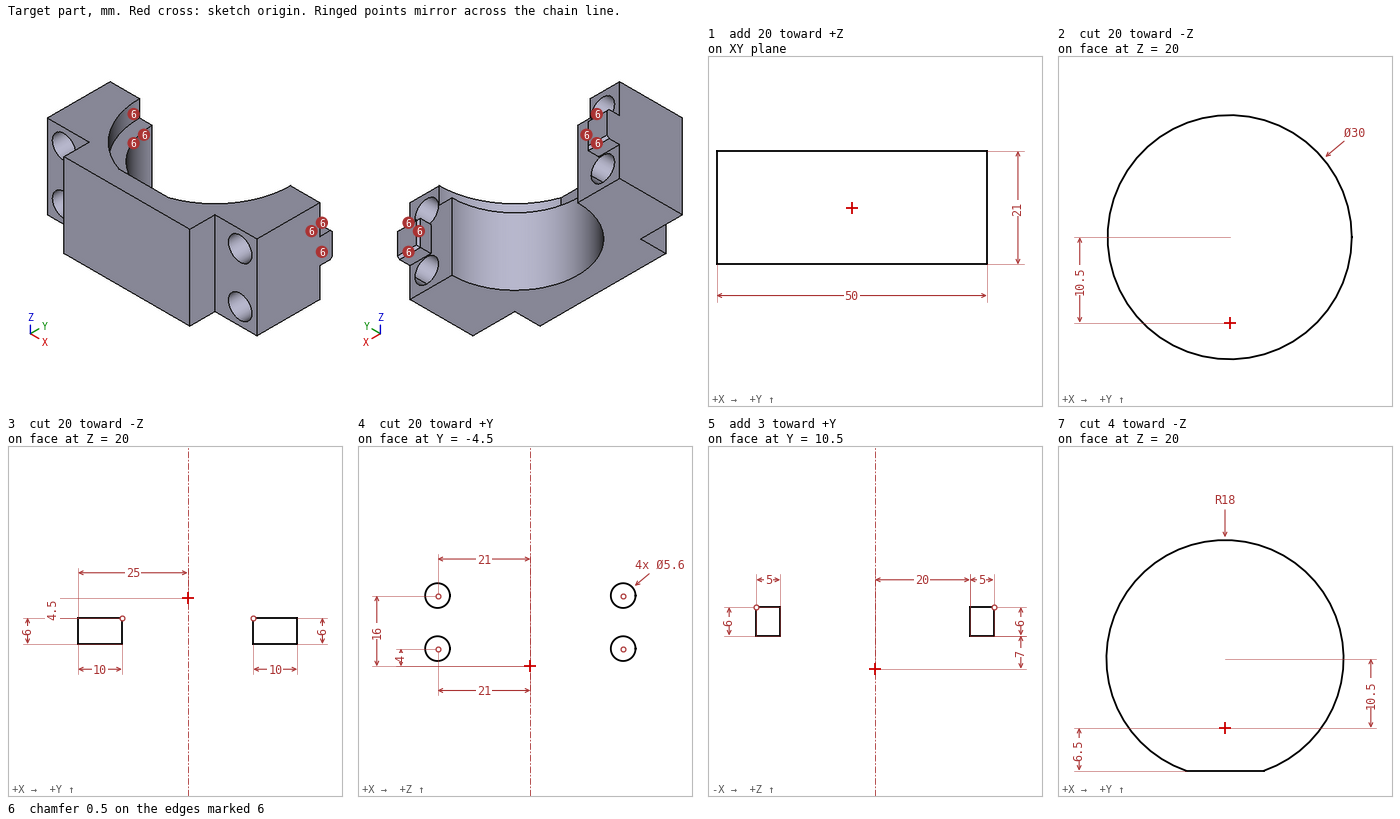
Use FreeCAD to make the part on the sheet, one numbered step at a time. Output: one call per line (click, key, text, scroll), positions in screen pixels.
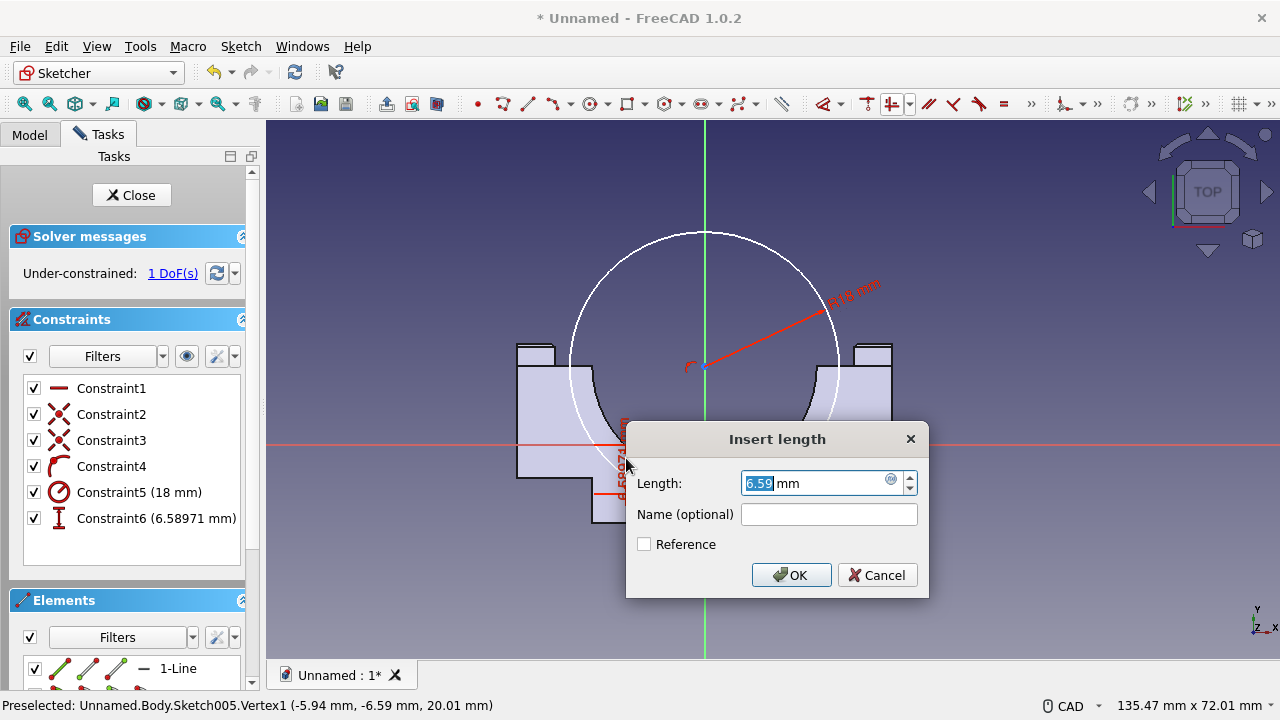
text(6.5)
key(Return)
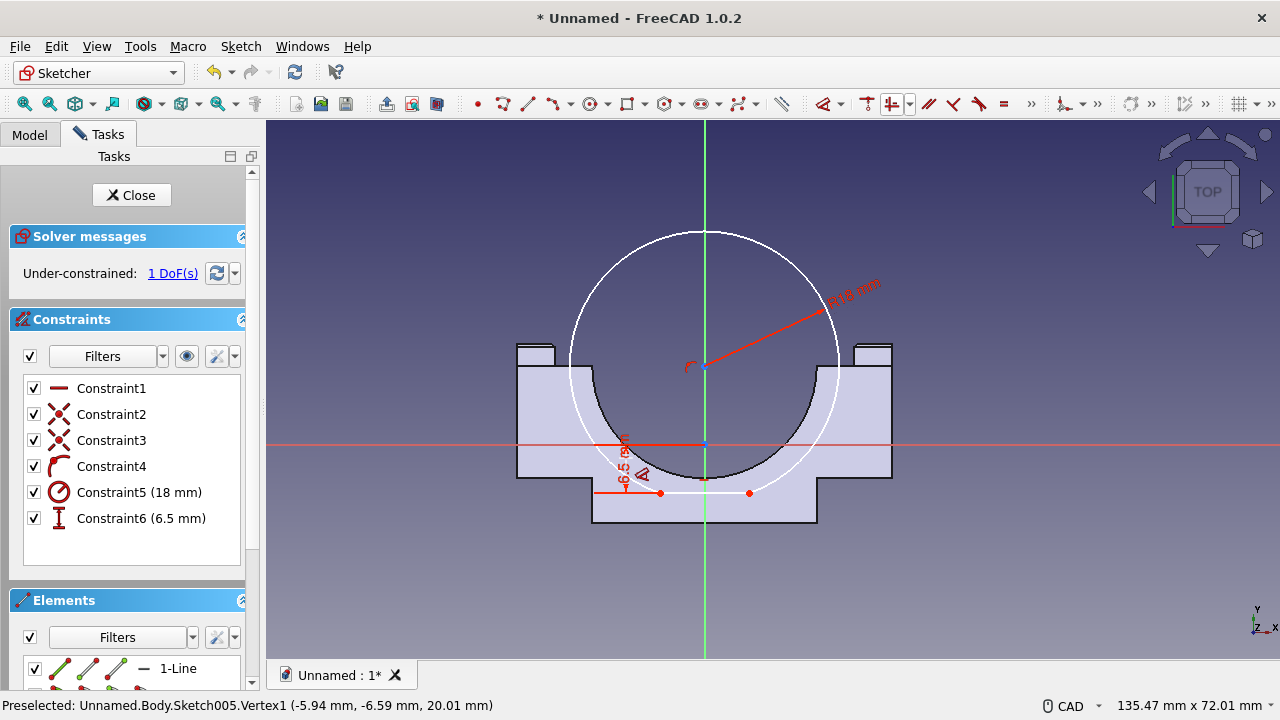
click(705, 366)
click(739, 405)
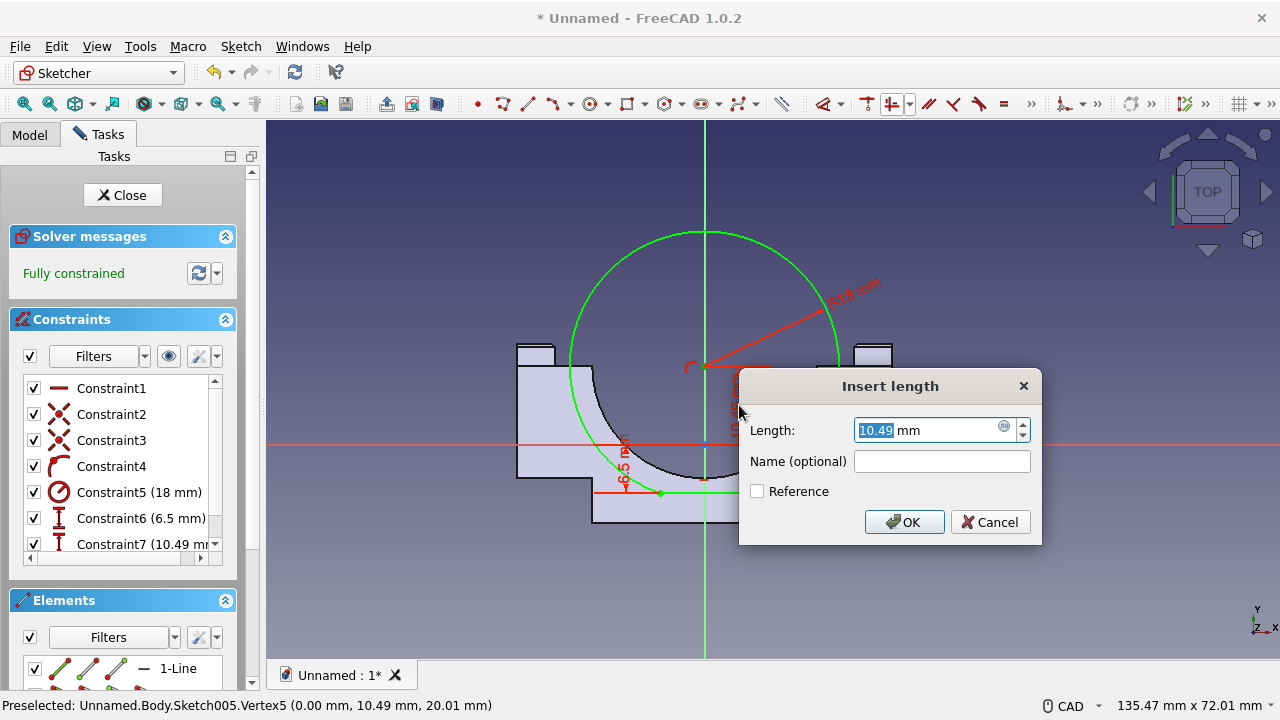
text(10.5)
key(Return)
key(Escape)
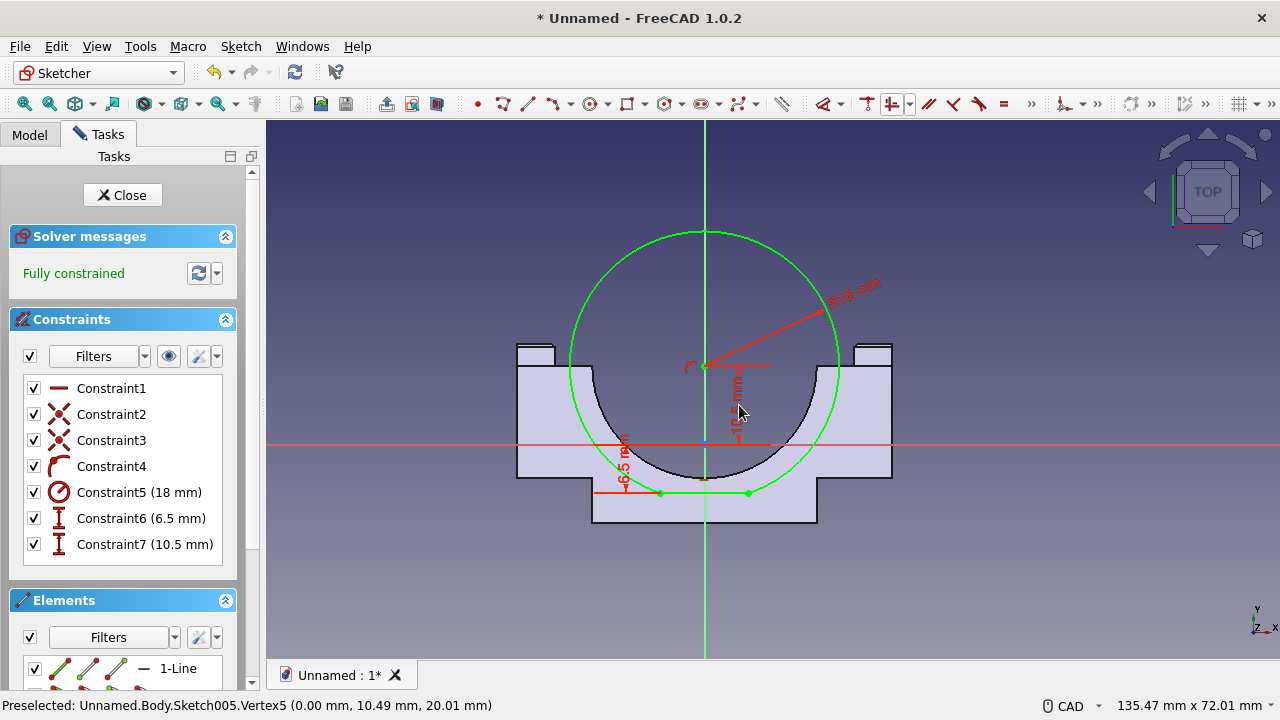
click(123, 195)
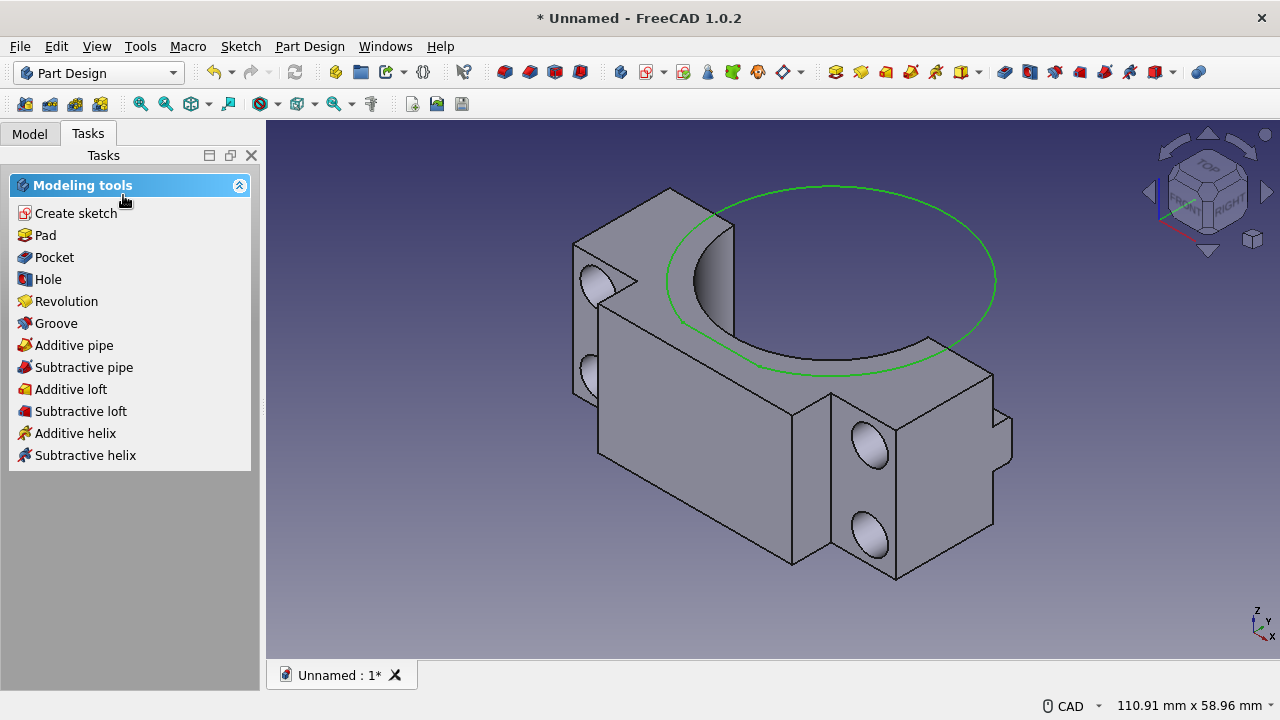
click(1005, 72)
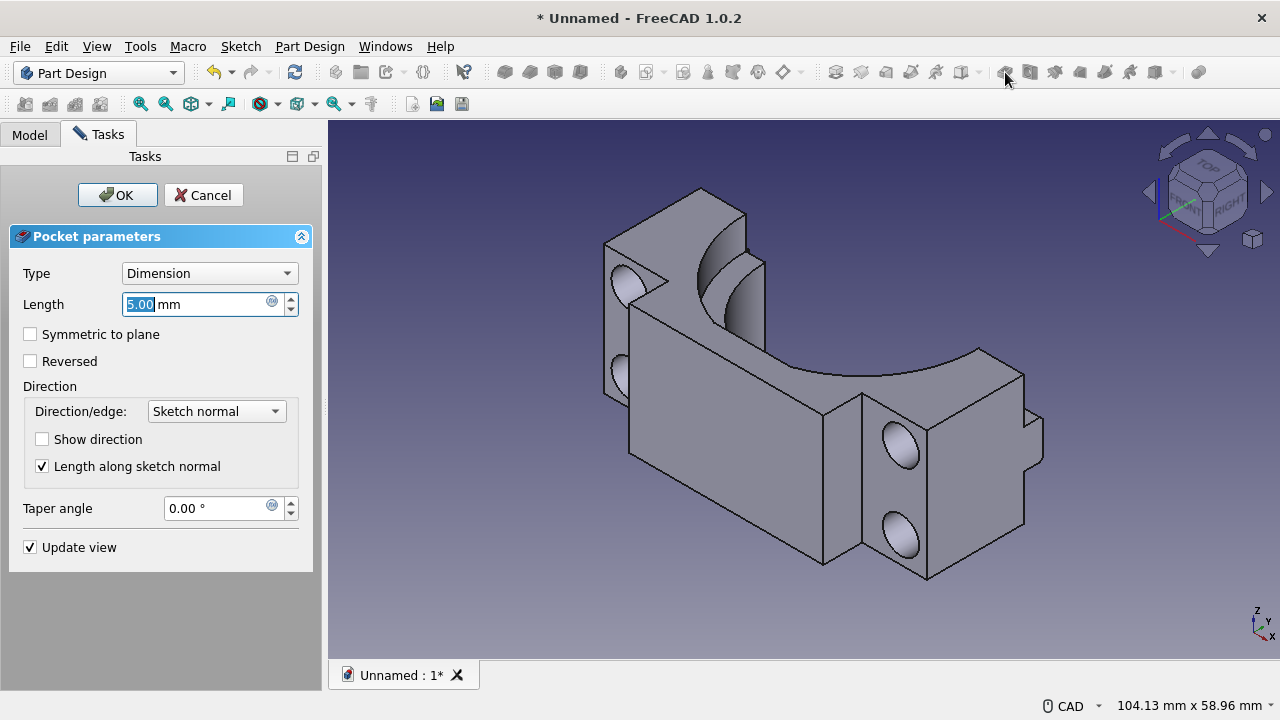
text(4)
key(Tab)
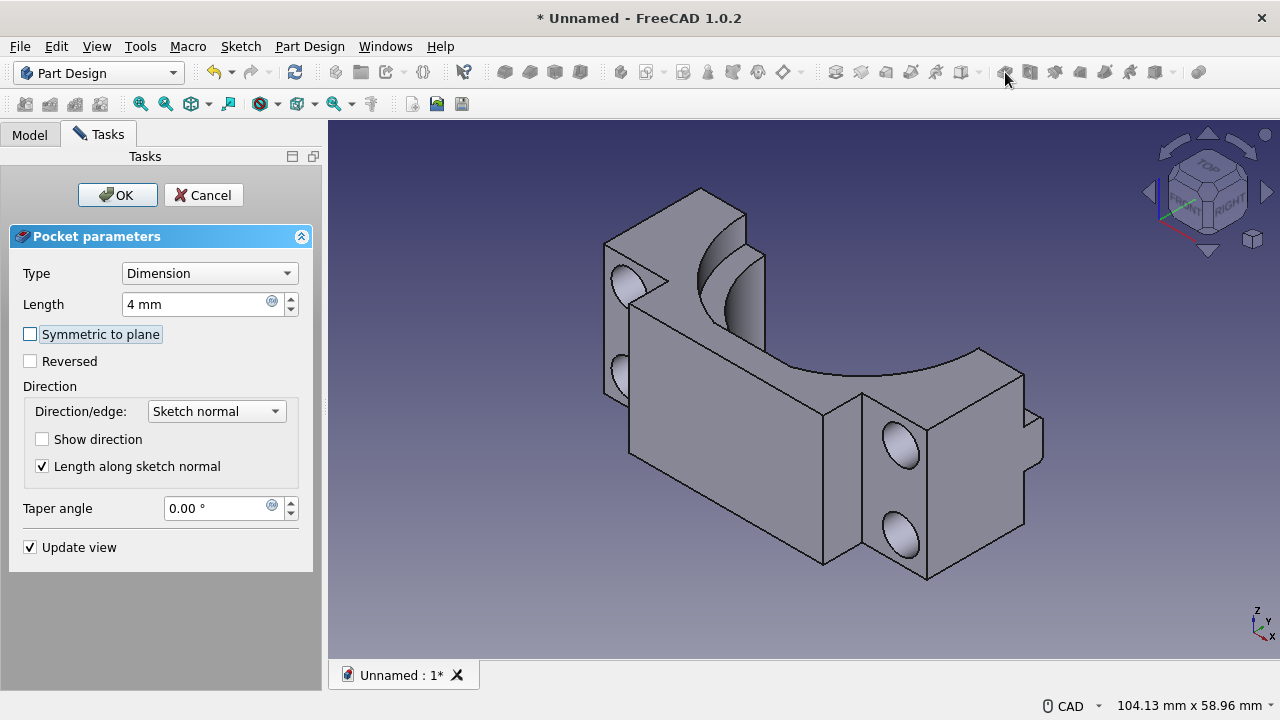
click(118, 195)